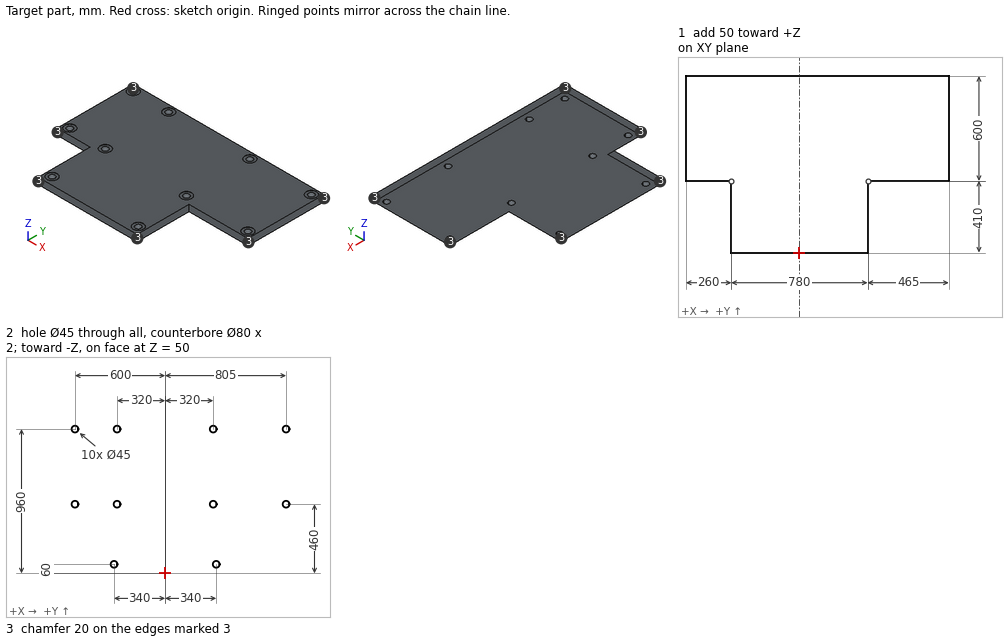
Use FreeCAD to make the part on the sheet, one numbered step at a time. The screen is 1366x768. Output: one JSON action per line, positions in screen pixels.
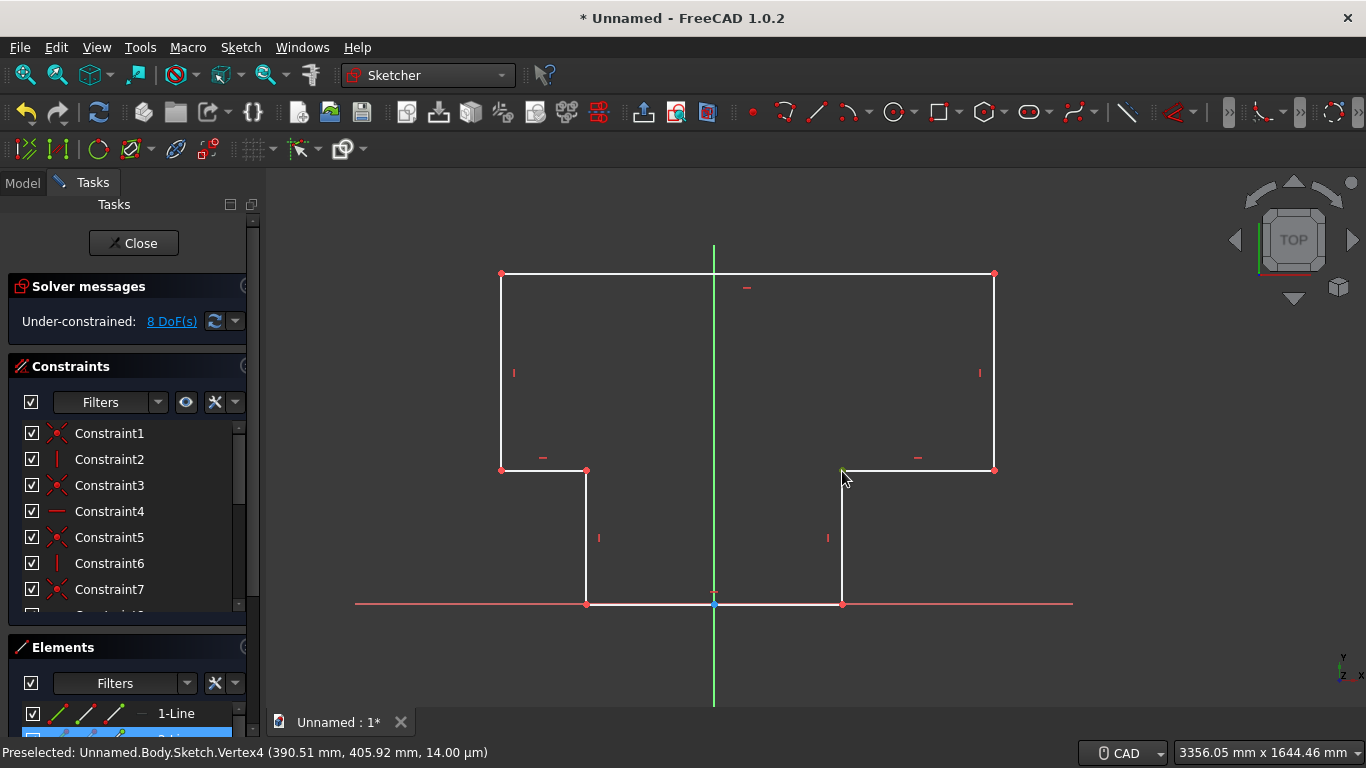
{"action": "left_click", "coordinate": [586, 471]}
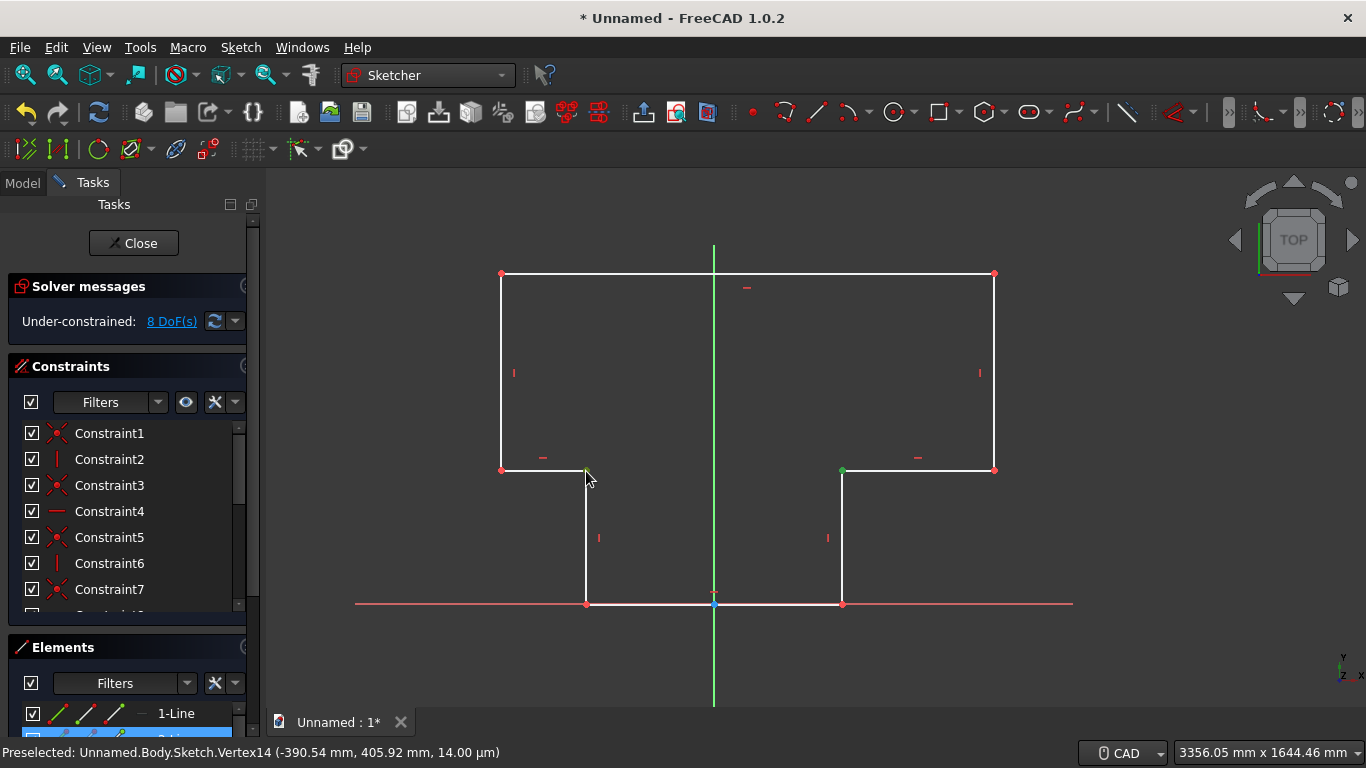
{"action": "left_click", "coordinate": [714, 644]}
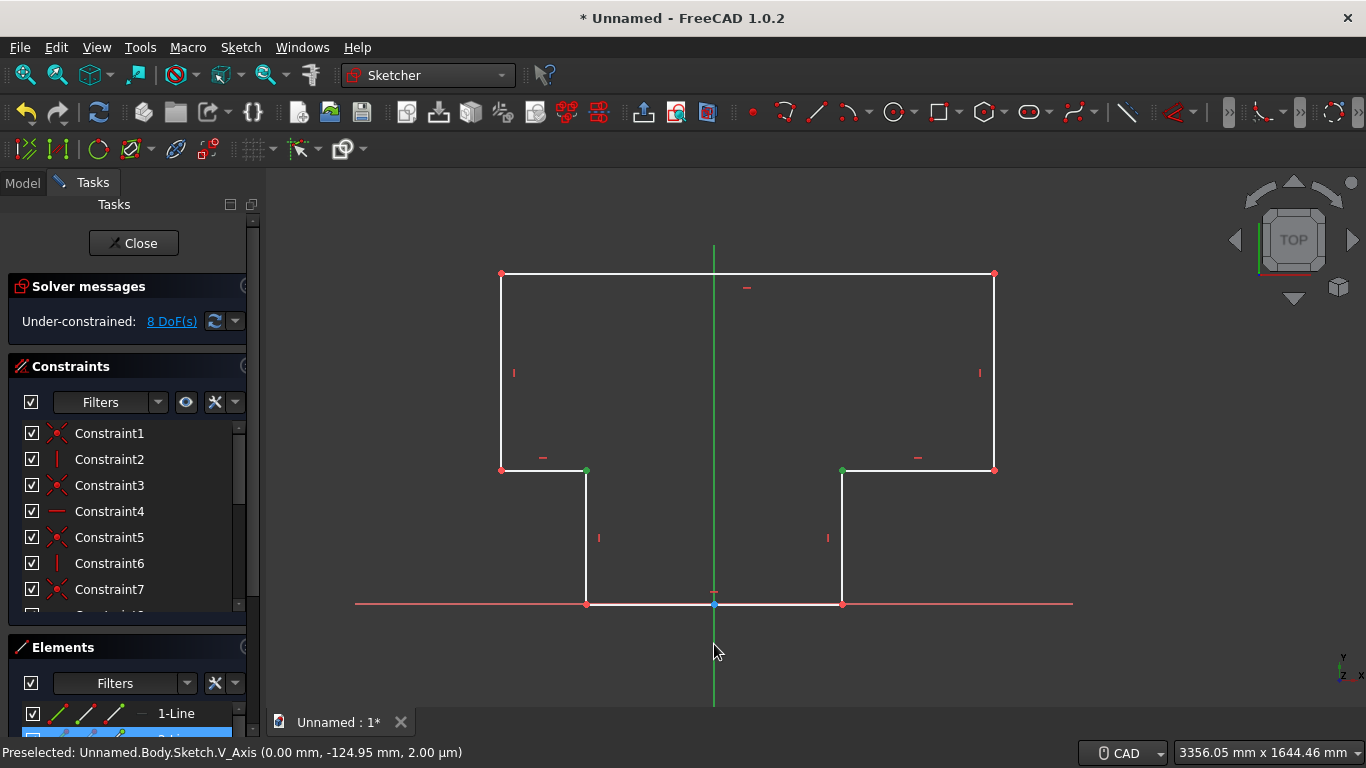
{"action": "key", "text": "s"}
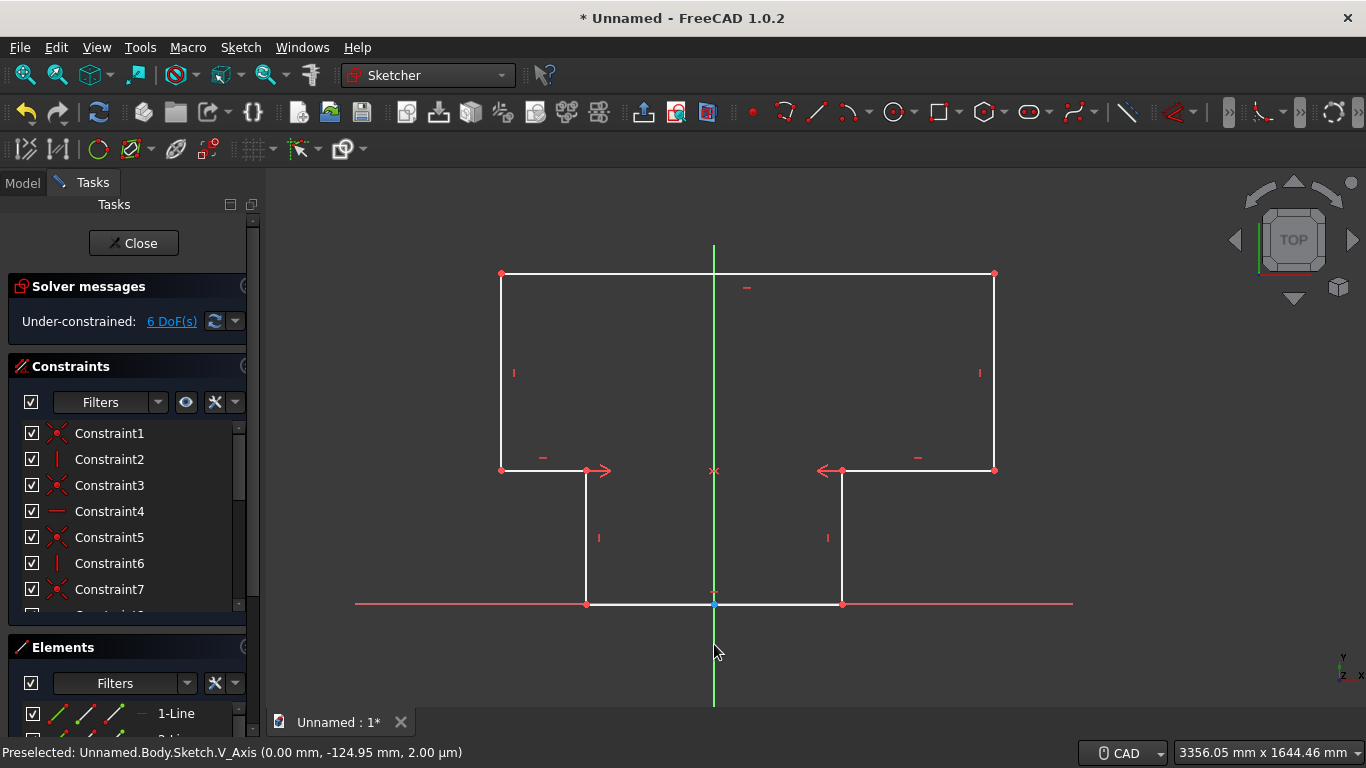
{"action": "left_click", "coordinate": [586, 605]}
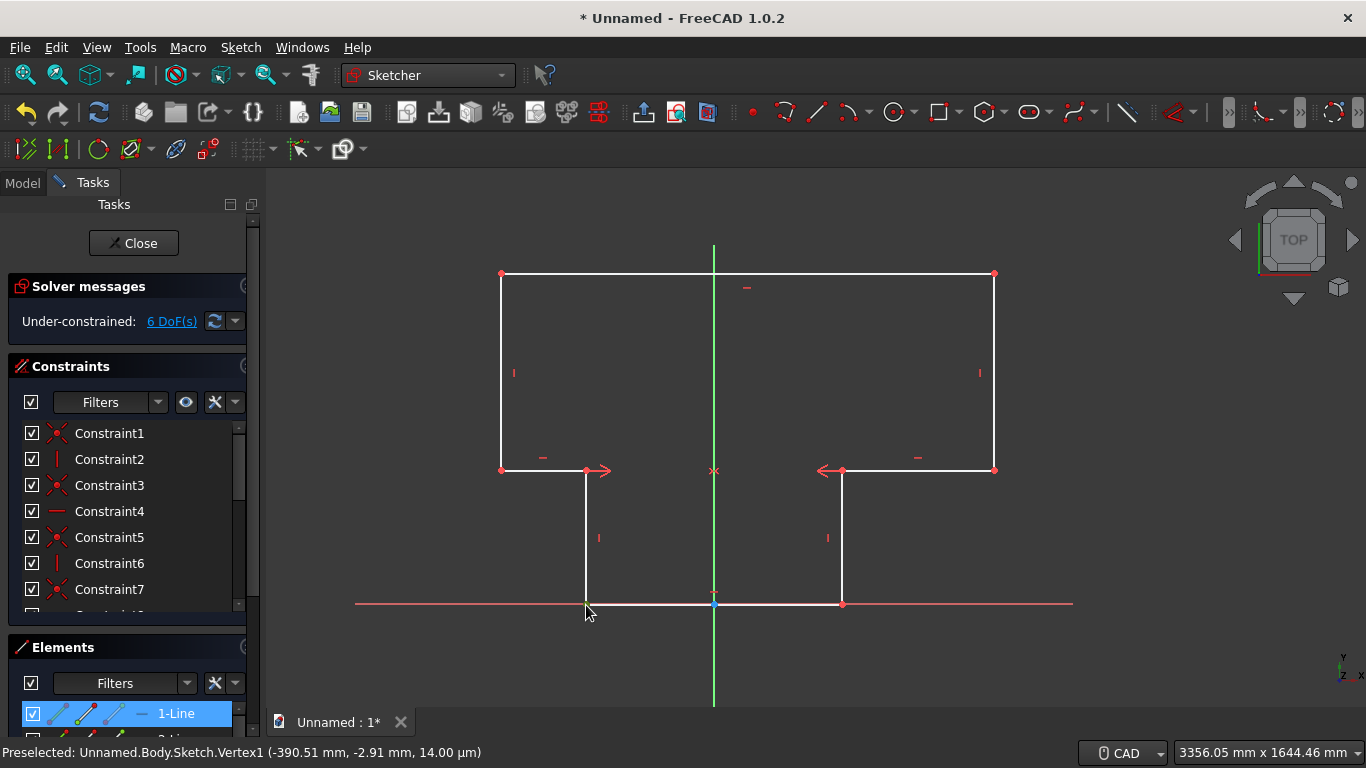
{"action": "left_click", "coordinate": [359, 604]}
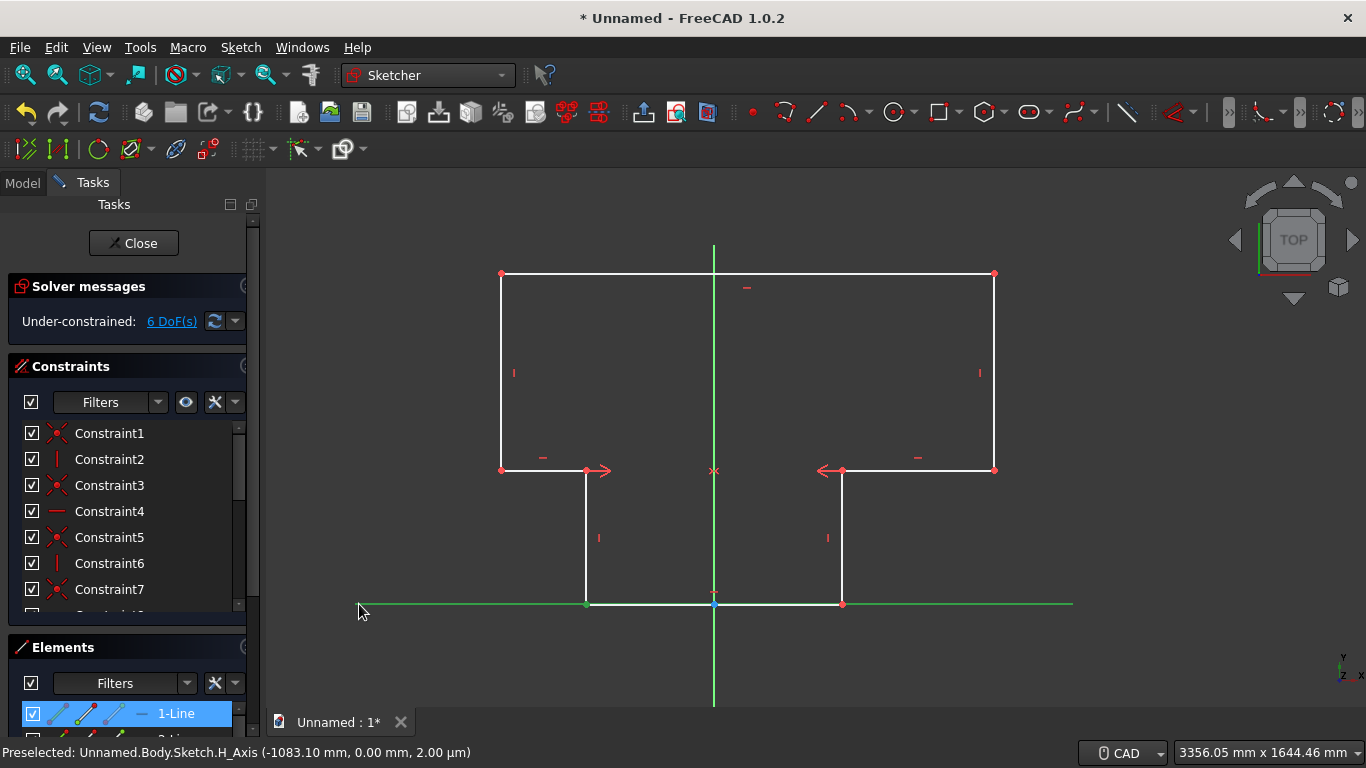
{"action": "key", "text": "c"}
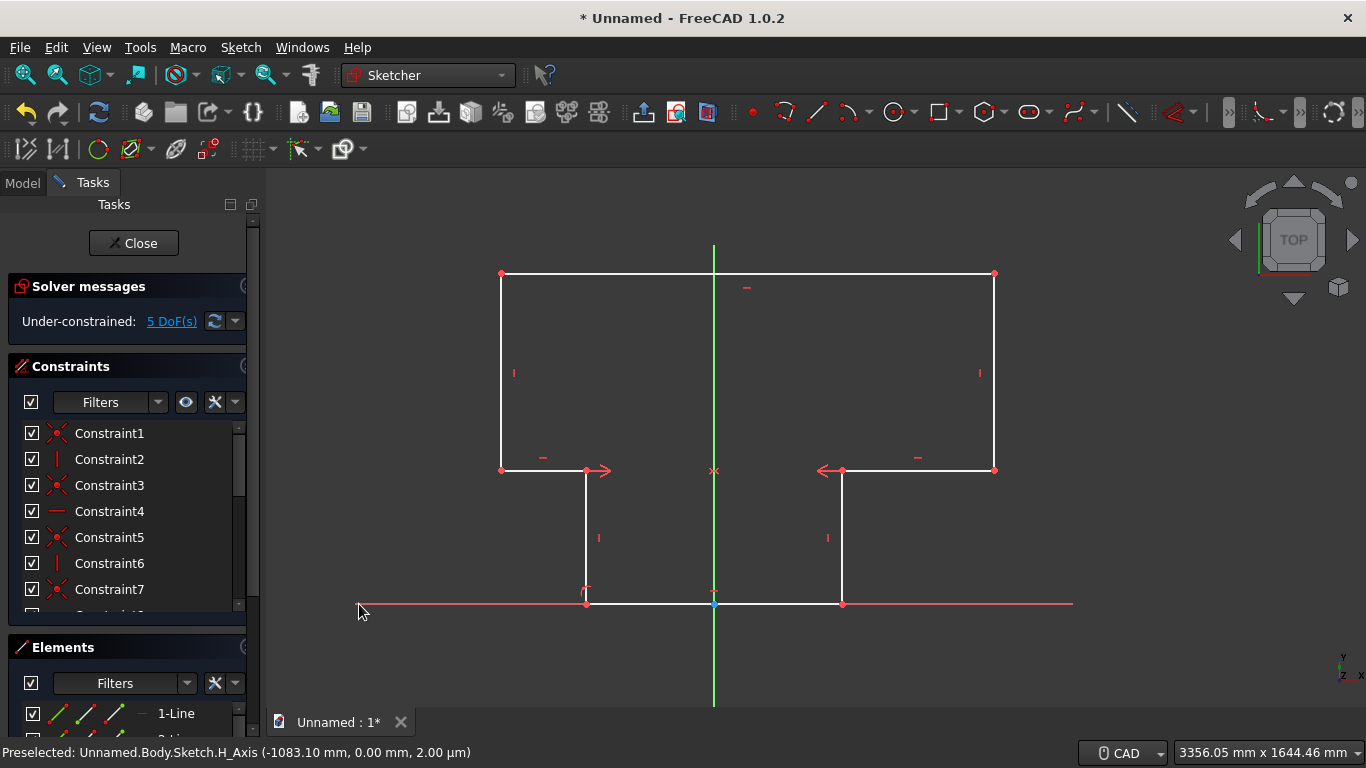
{"action": "left_click", "coordinate": [663, 604]}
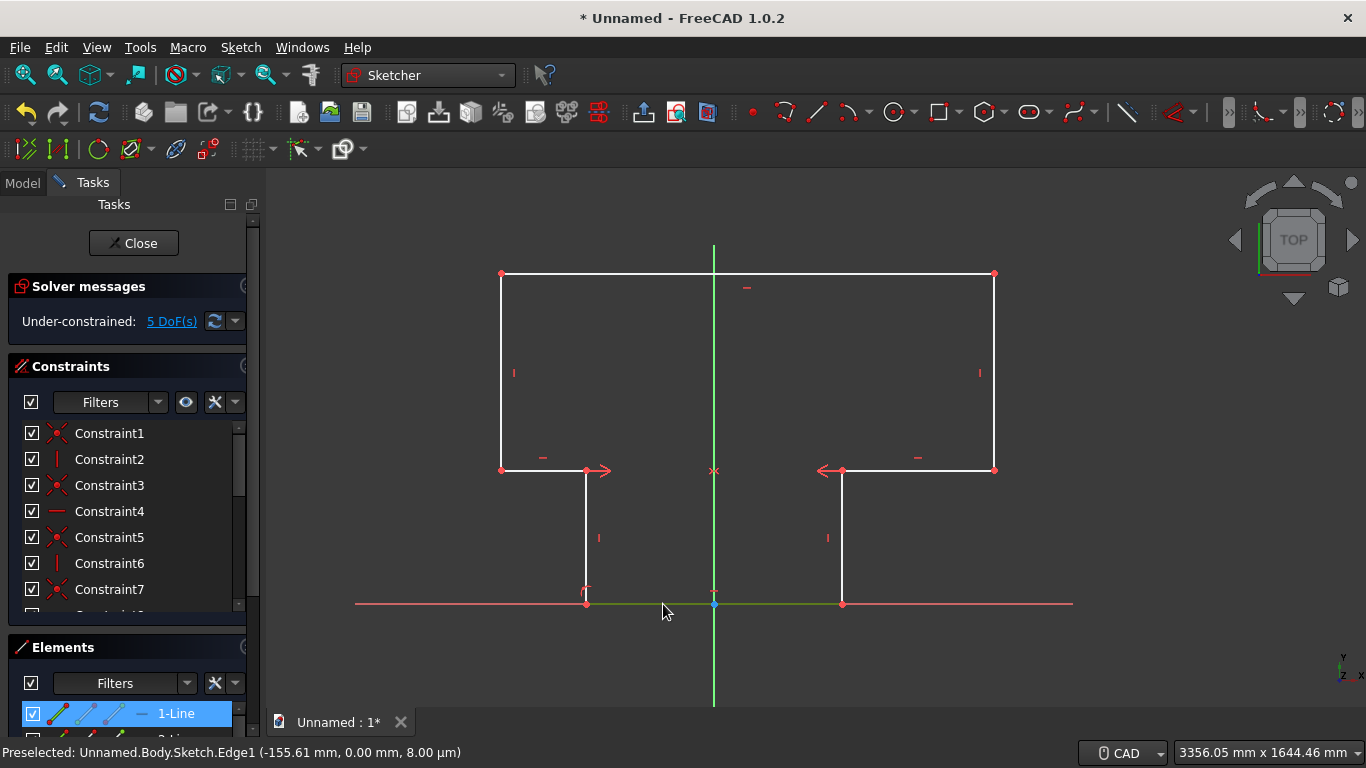
{"action": "key", "text": "l"}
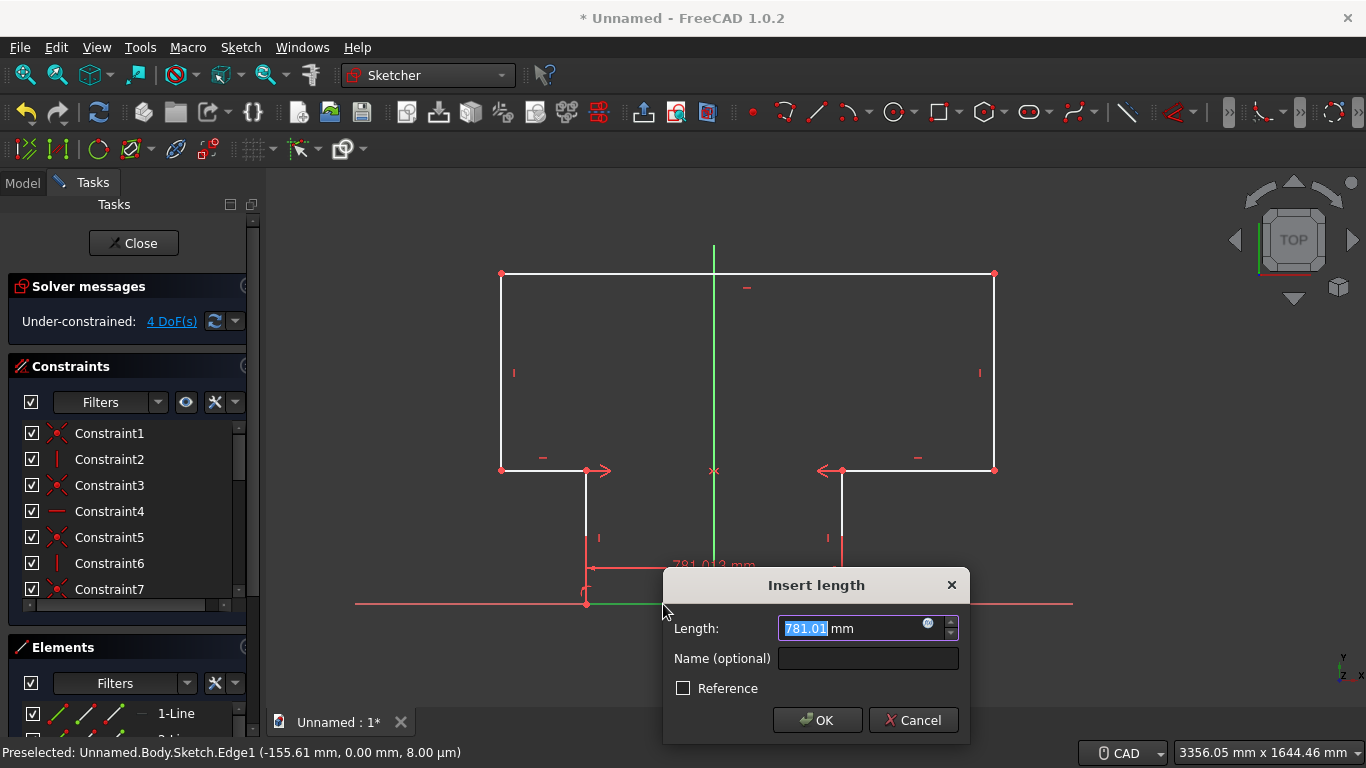
{"action": "type", "text": "780"}
{"action": "key", "text": "Return"}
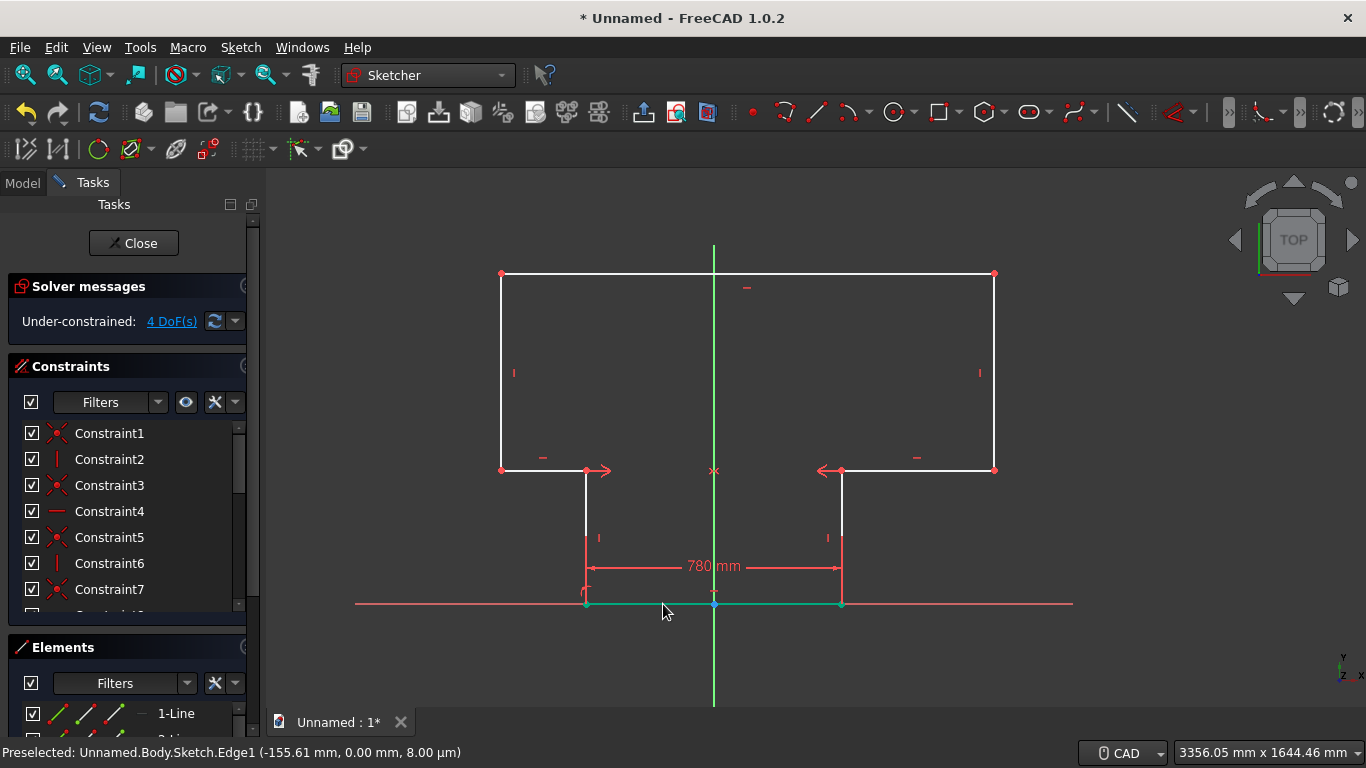
{"action": "left_click", "coordinate": [842, 564]}